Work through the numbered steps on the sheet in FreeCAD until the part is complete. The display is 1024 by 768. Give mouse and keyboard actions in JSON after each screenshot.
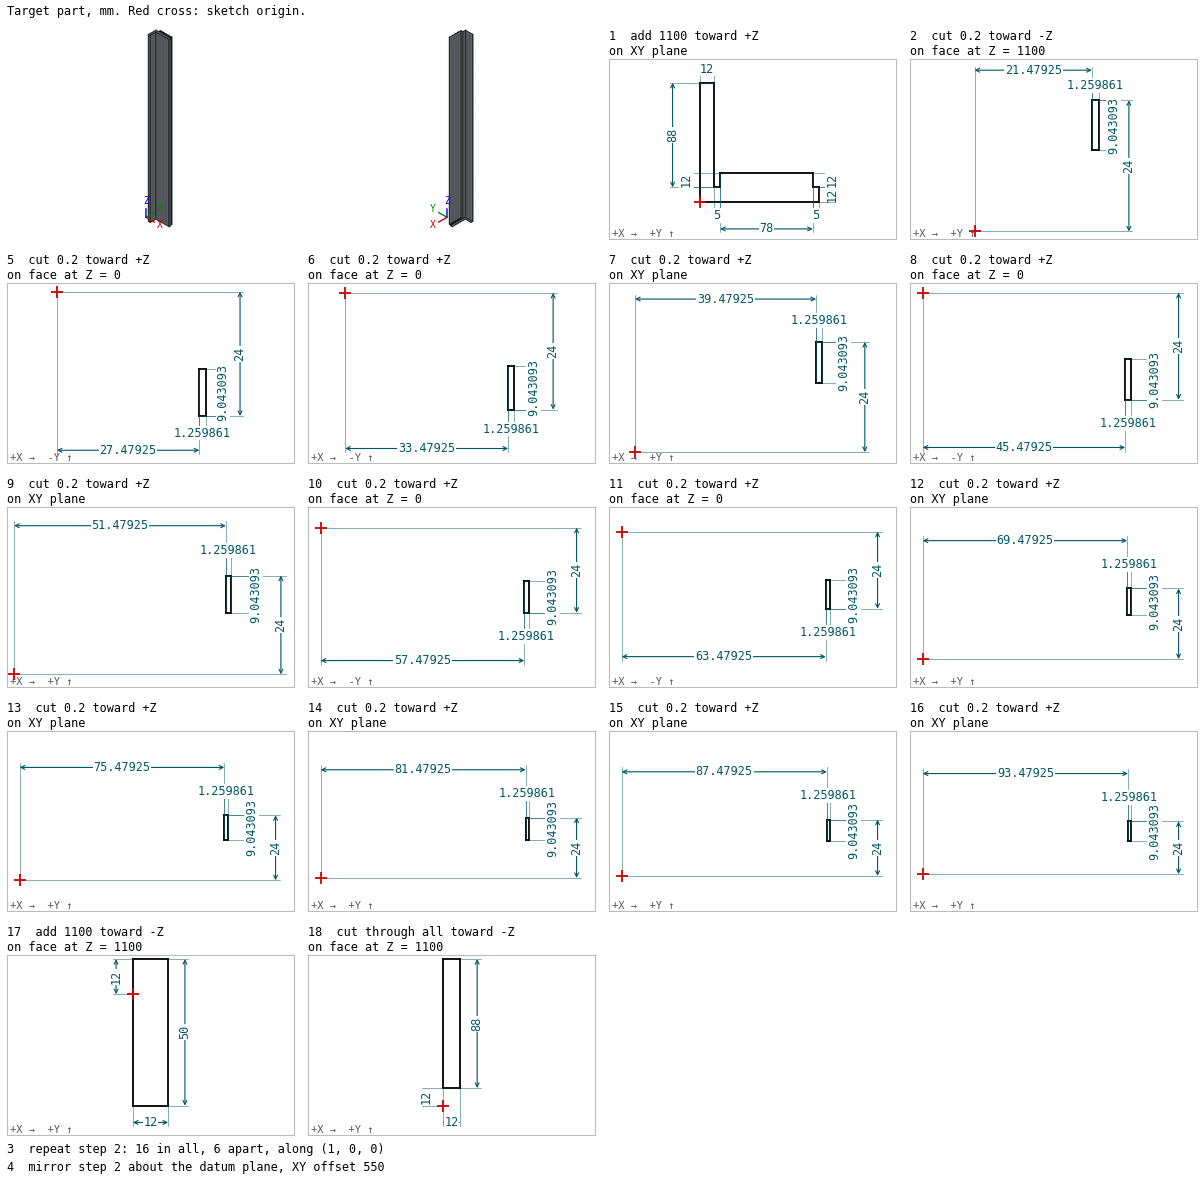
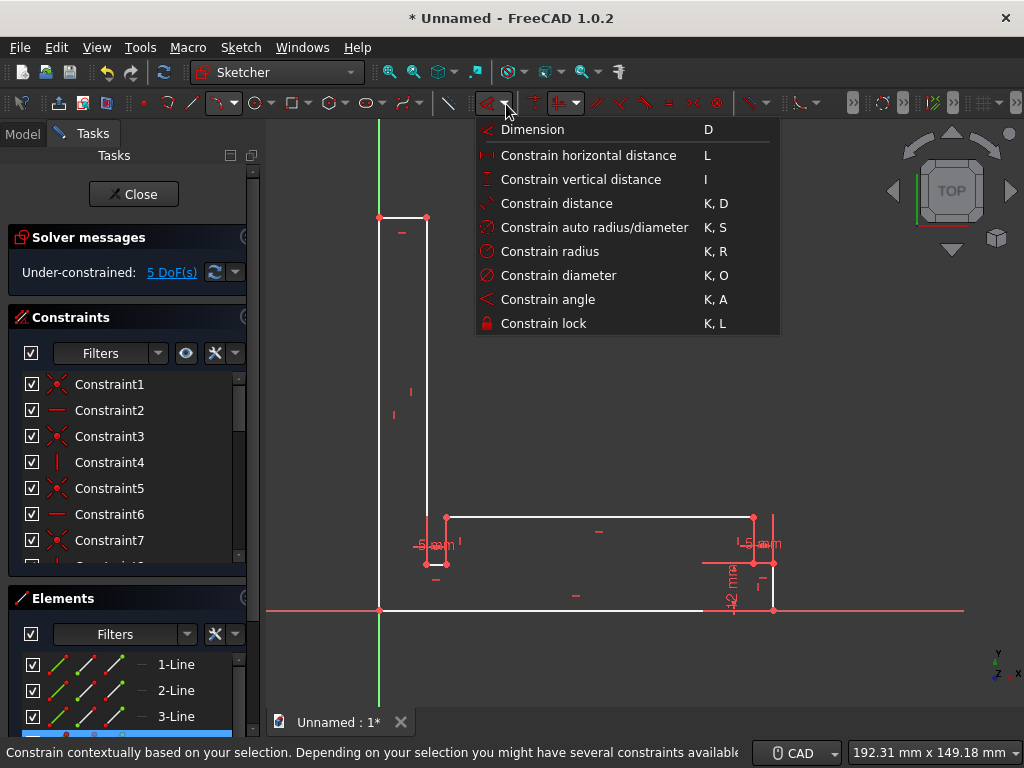
{"action": "left_click", "coordinate": [628, 179]}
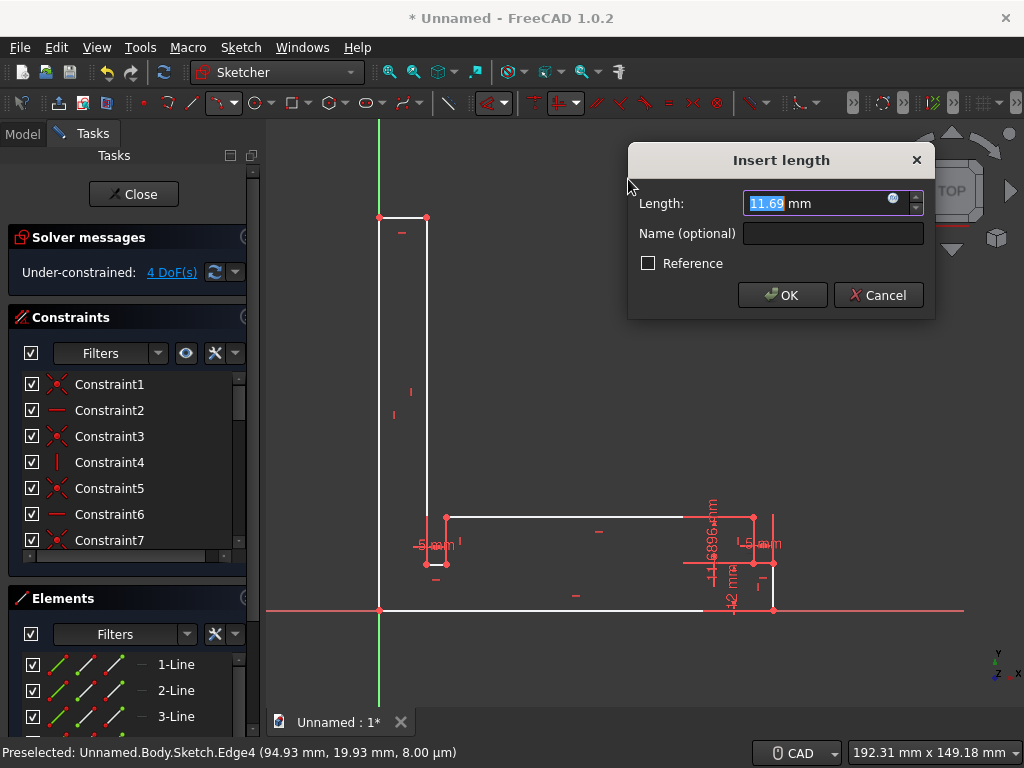
{"action": "type", "text": "12"}
{"action": "key", "text": "Return"}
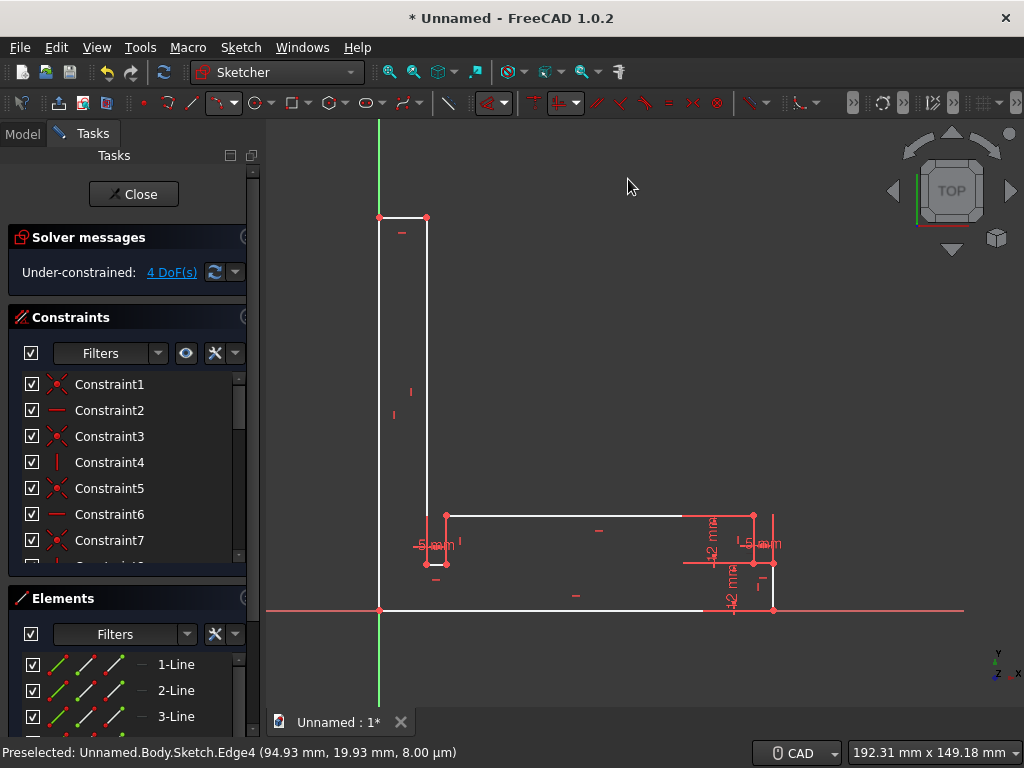
{"action": "left_click", "coordinate": [661, 516]}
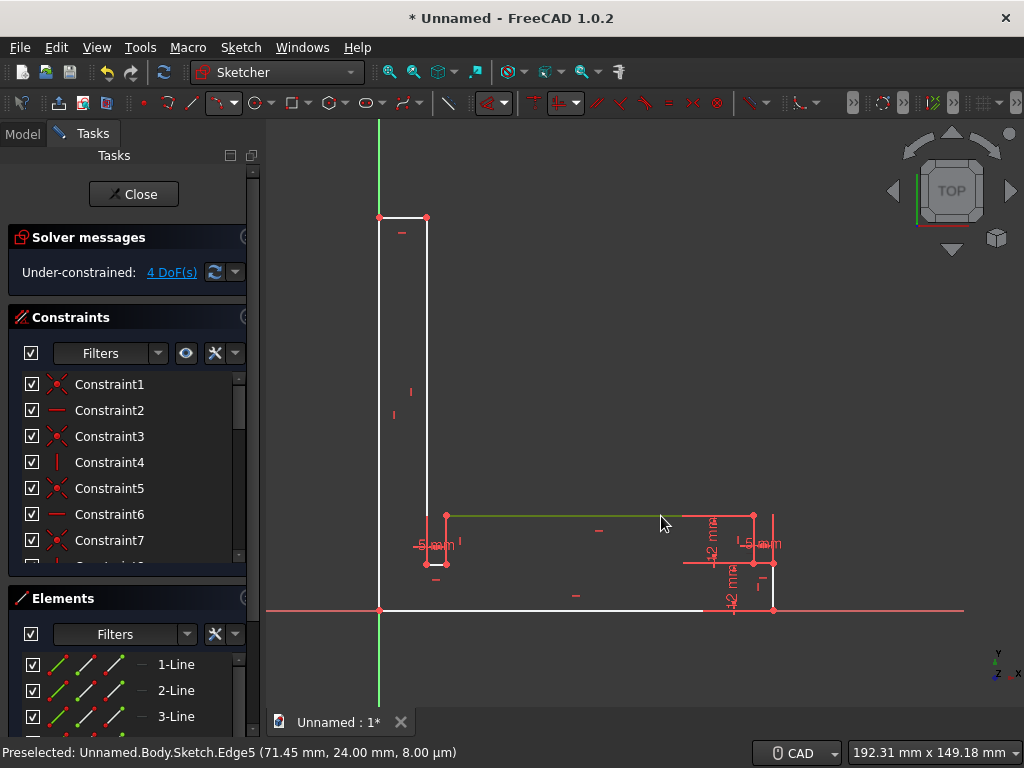
{"action": "left_click", "coordinate": [506, 104]}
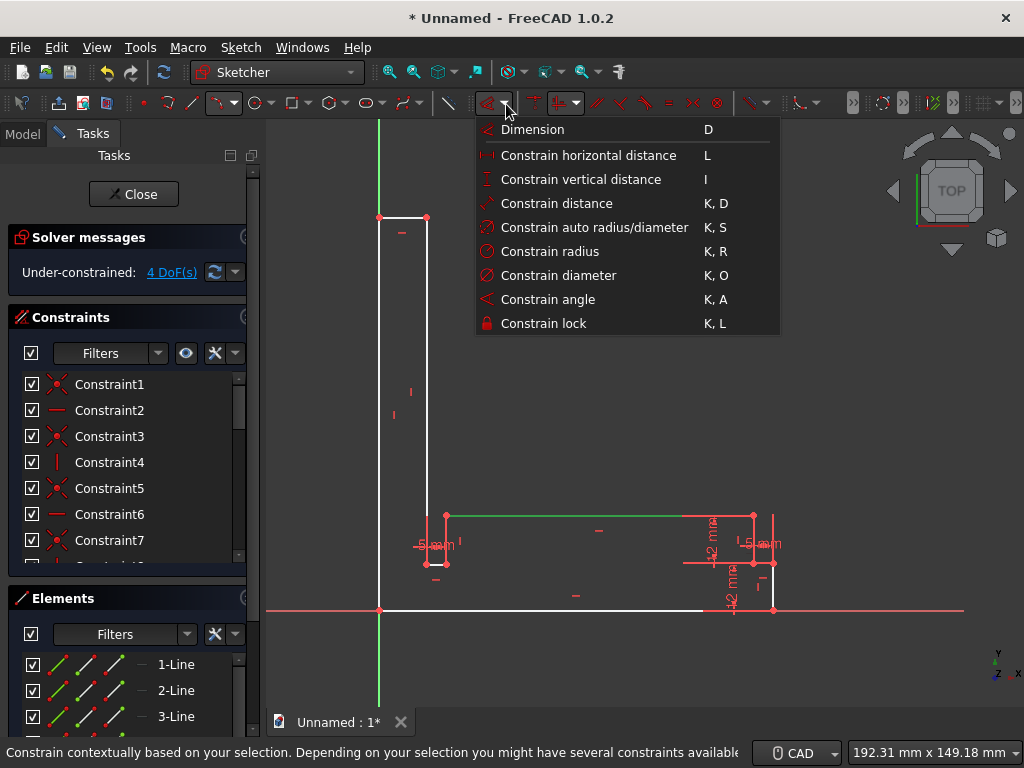
{"action": "left_click", "coordinate": [628, 155]}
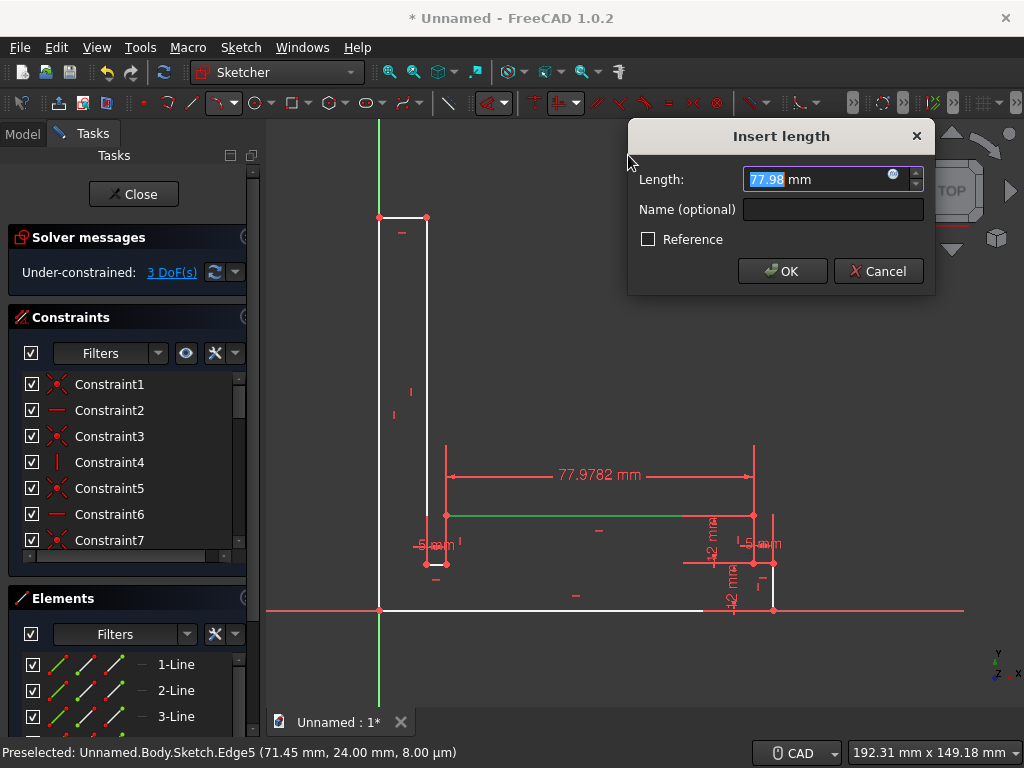
{"action": "type", "text": "78"}
{"action": "key", "text": "Return"}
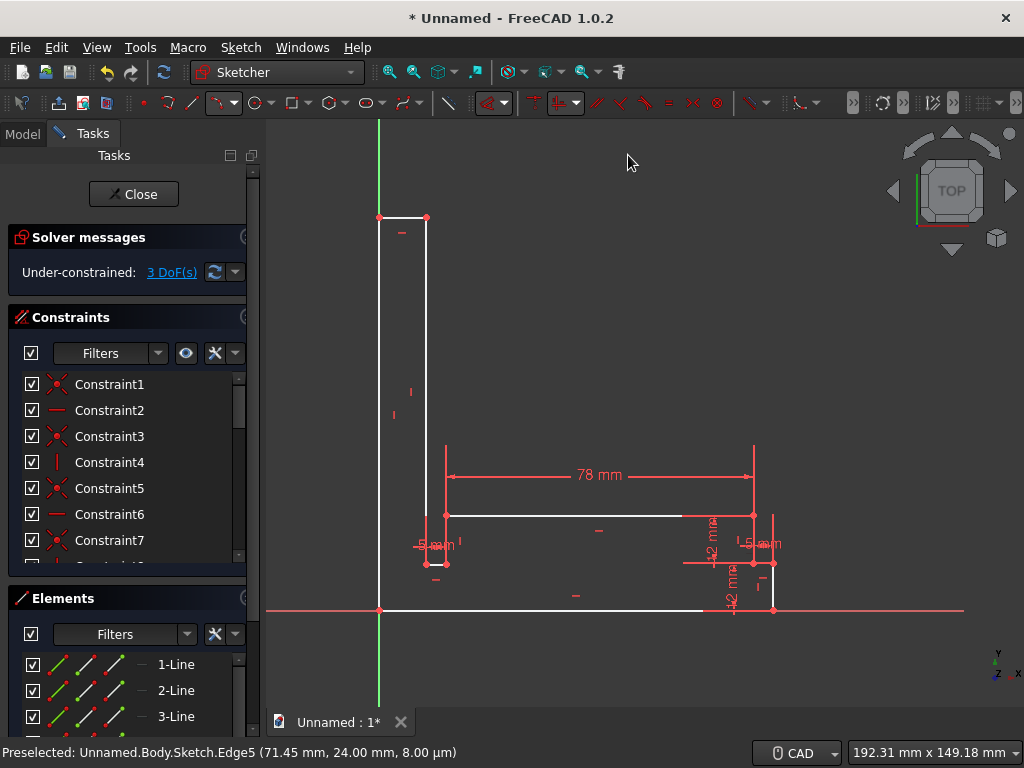
{"action": "left_click", "coordinate": [446, 531]}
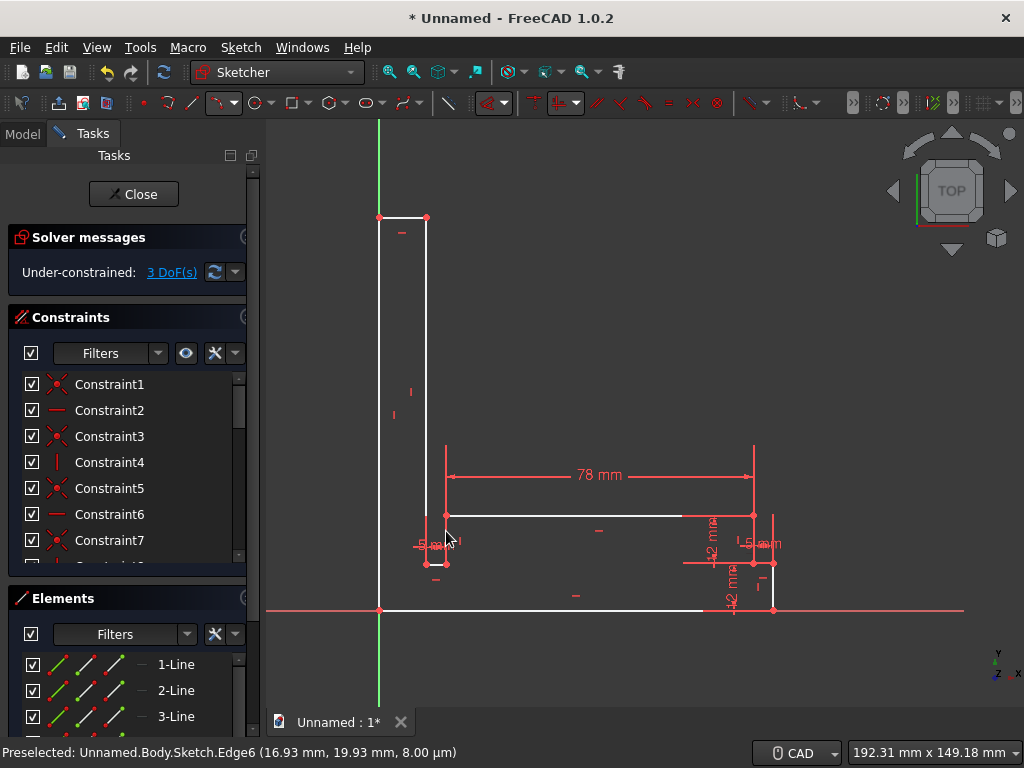
{"action": "left_click", "coordinate": [506, 104]}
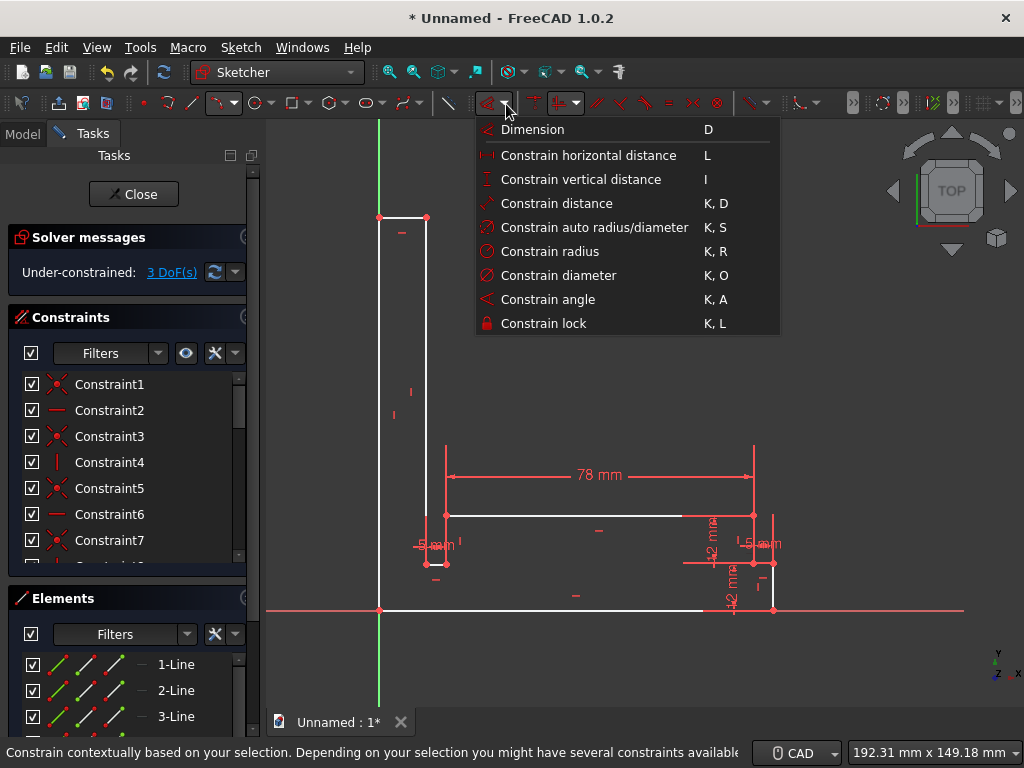
{"action": "left_click", "coordinate": [628, 179]}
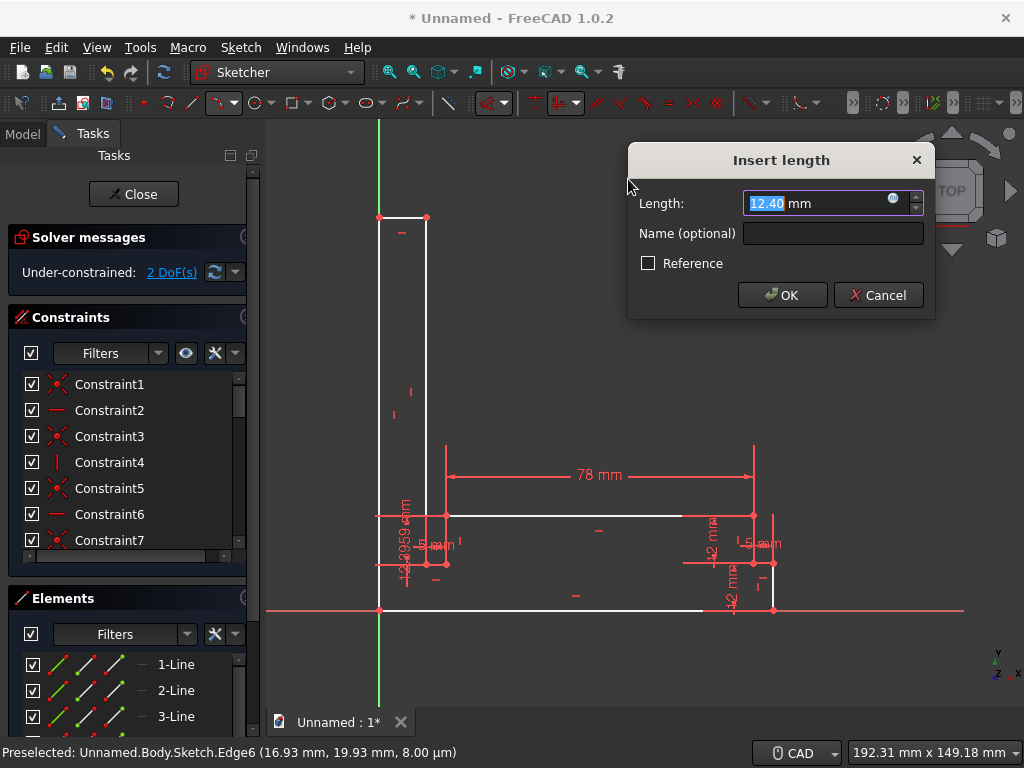
{"action": "type", "text": "12"}
{"action": "key", "text": "Return"}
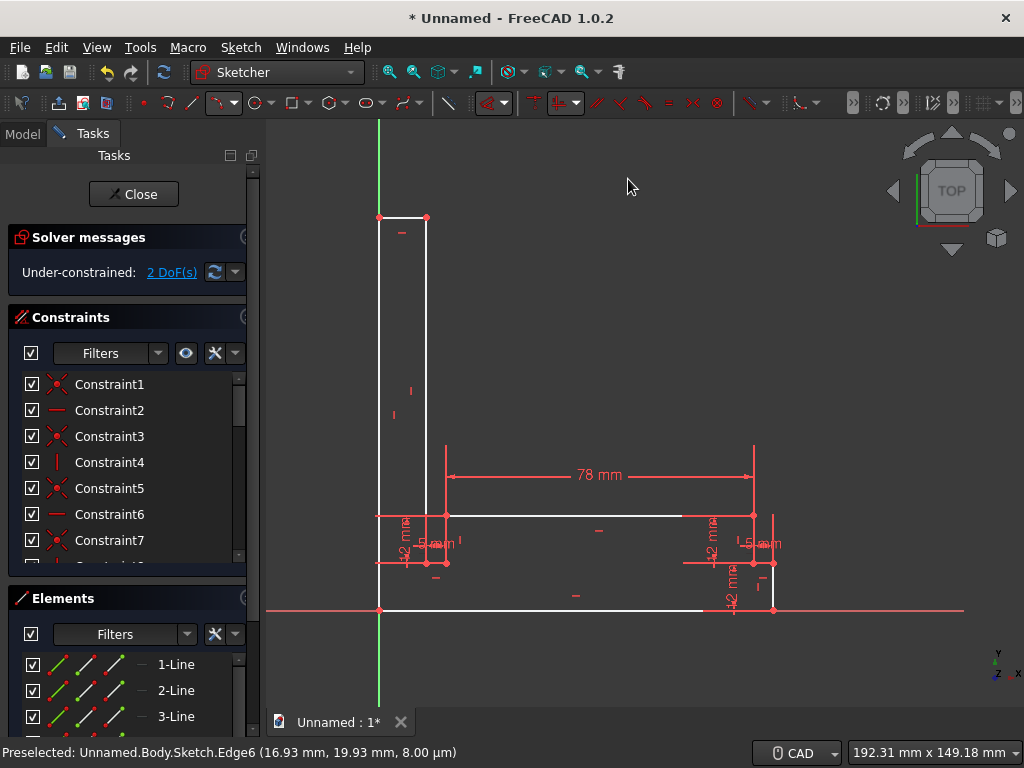
{"action": "left_click", "coordinate": [426, 460]}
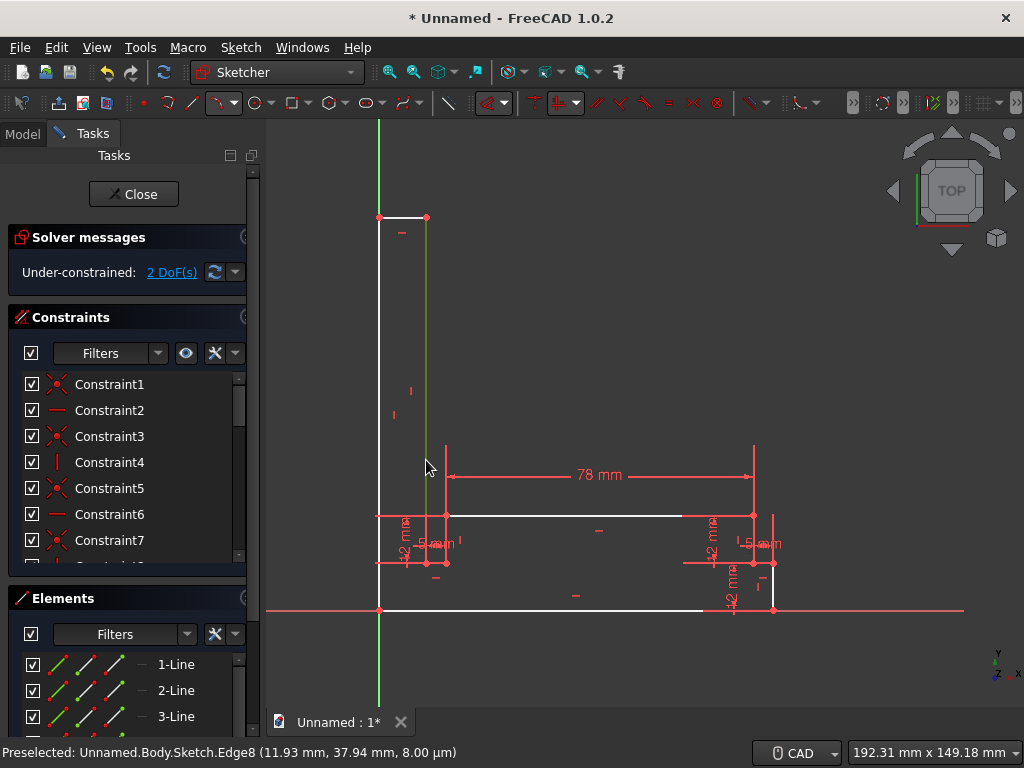
{"action": "key", "text": "i"}